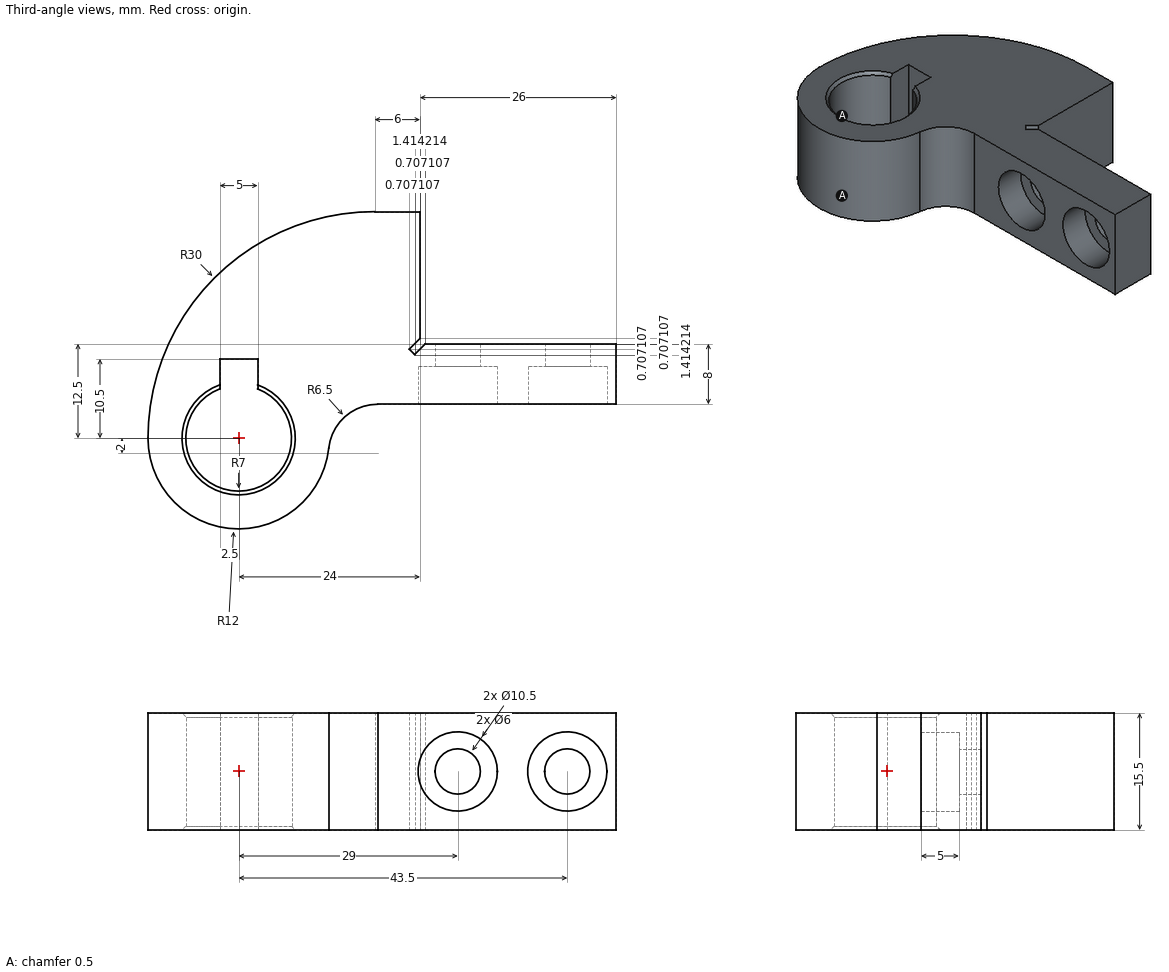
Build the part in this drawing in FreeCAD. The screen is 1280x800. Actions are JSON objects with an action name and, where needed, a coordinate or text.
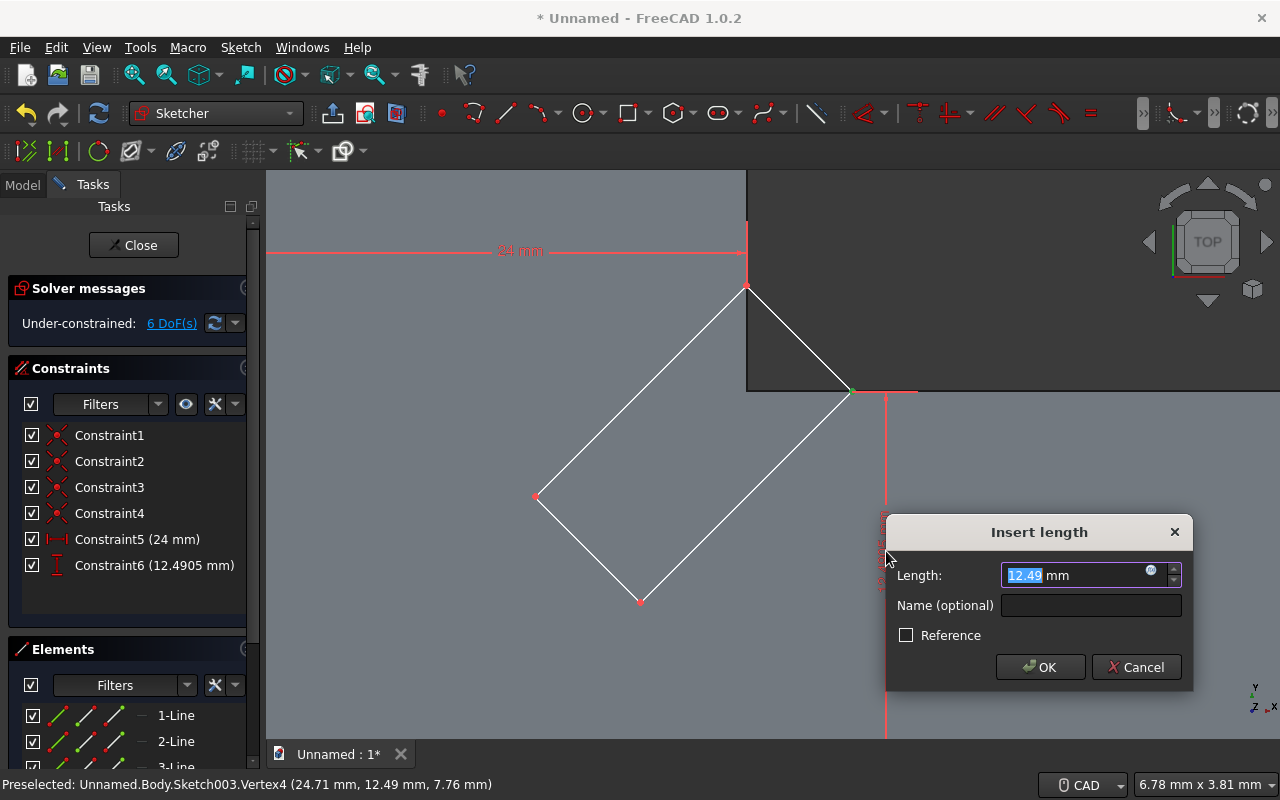
{"action": "type", "text": "12.5"}
{"action": "key", "text": "Return"}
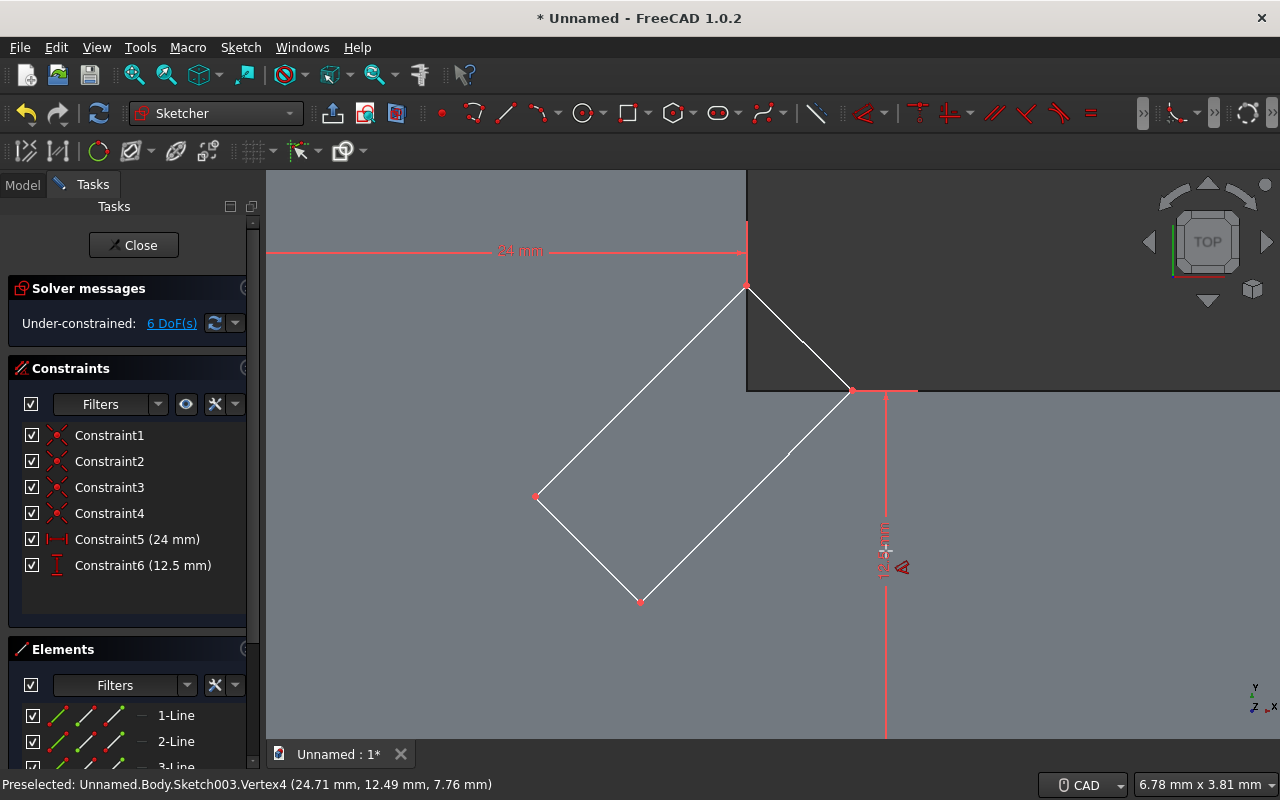
{"action": "left_click", "coordinate": [567, 529]}
{"action": "left_click", "coordinate": [588, 637]}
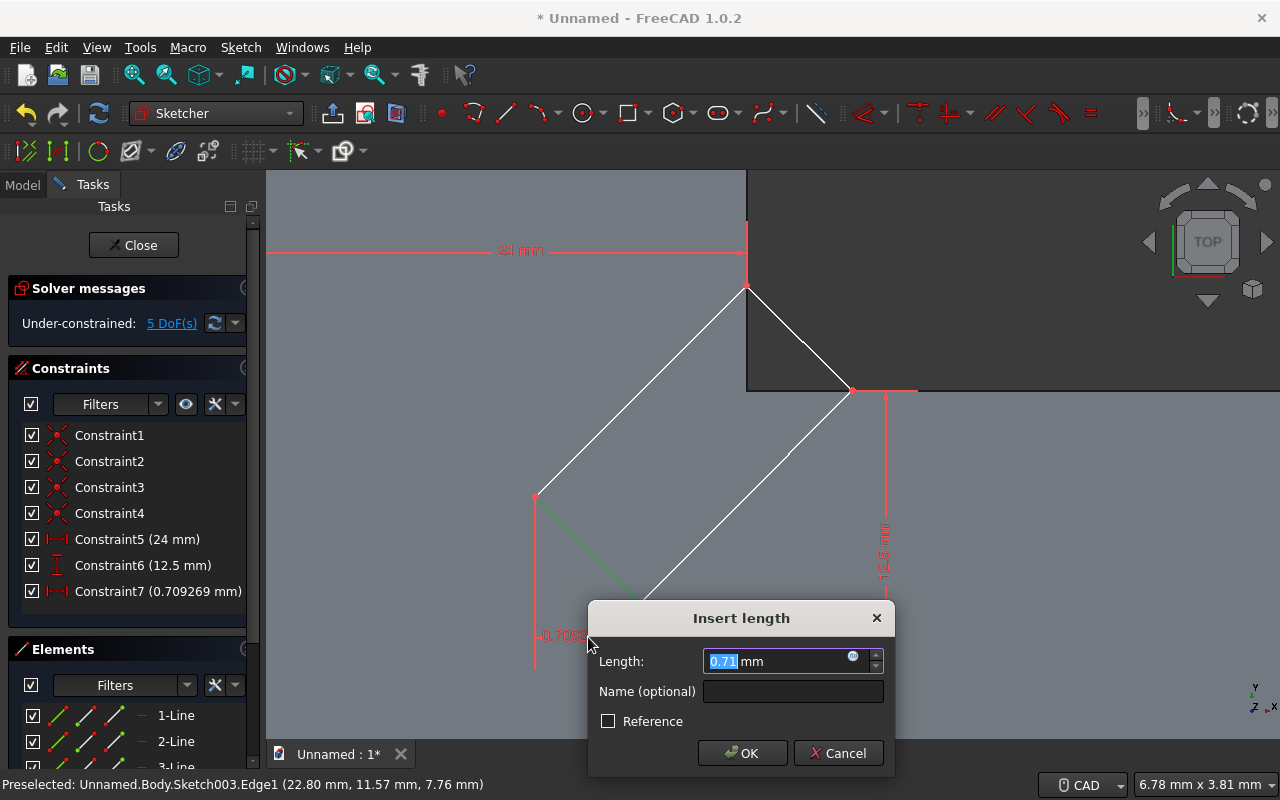
{"action": "type", "text": "0.707107"}
{"action": "key", "text": "Return"}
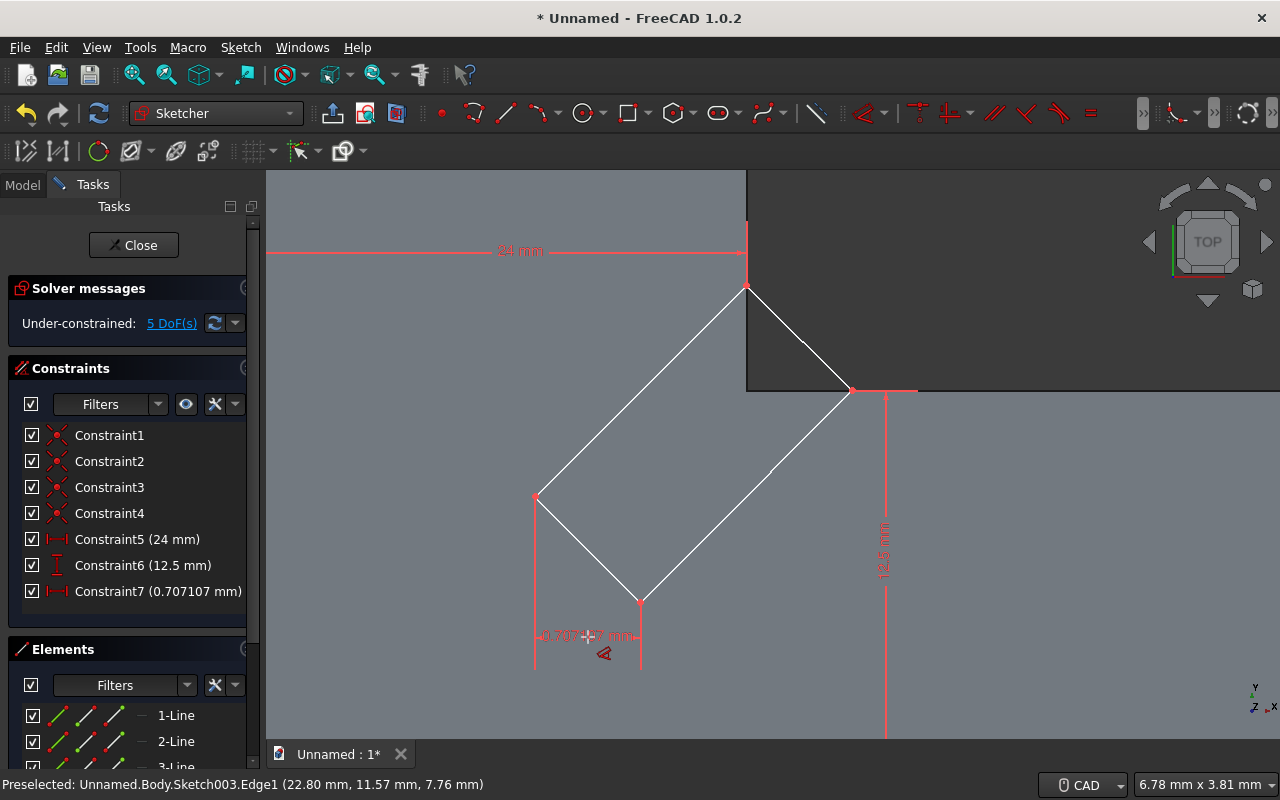
{"action": "left_click", "coordinate": [567, 529]}
{"action": "left_click", "coordinate": [501, 550]}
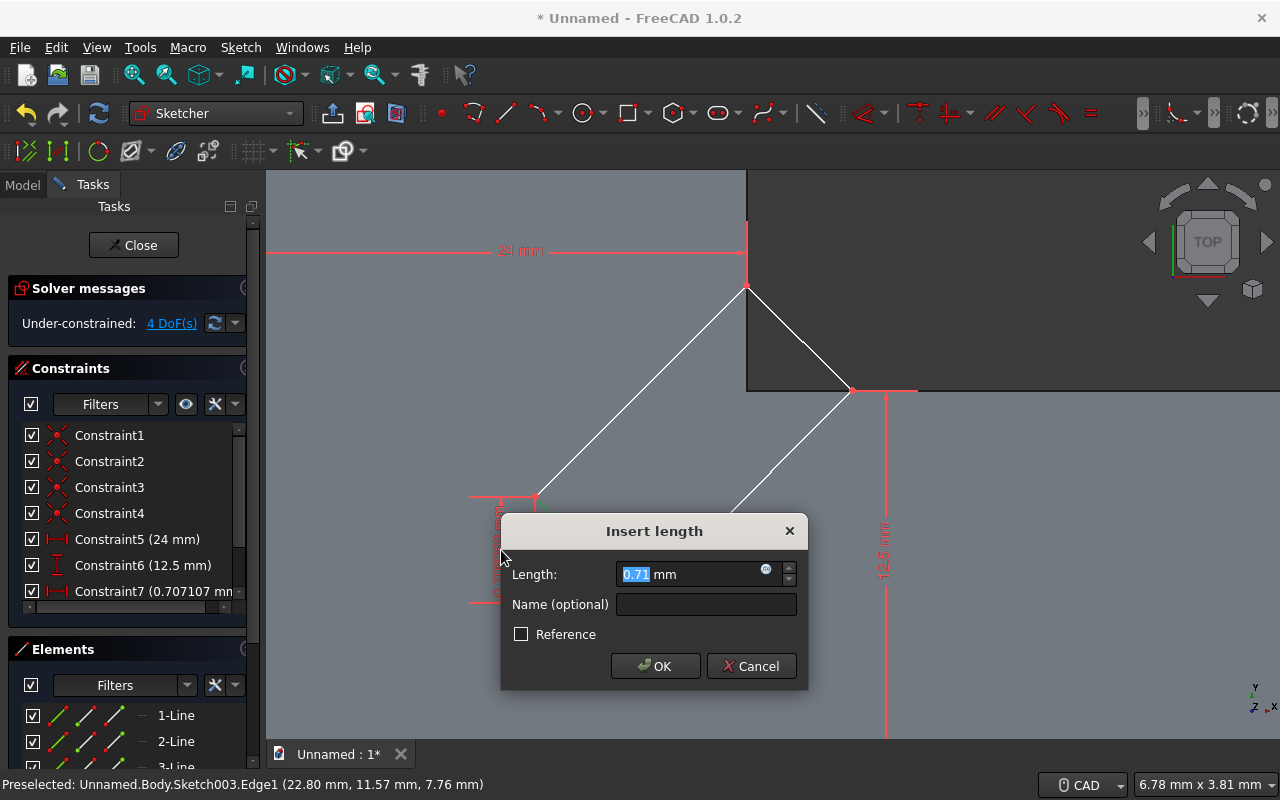
{"action": "type", "text": "0.707107"}
{"action": "key", "text": "Return"}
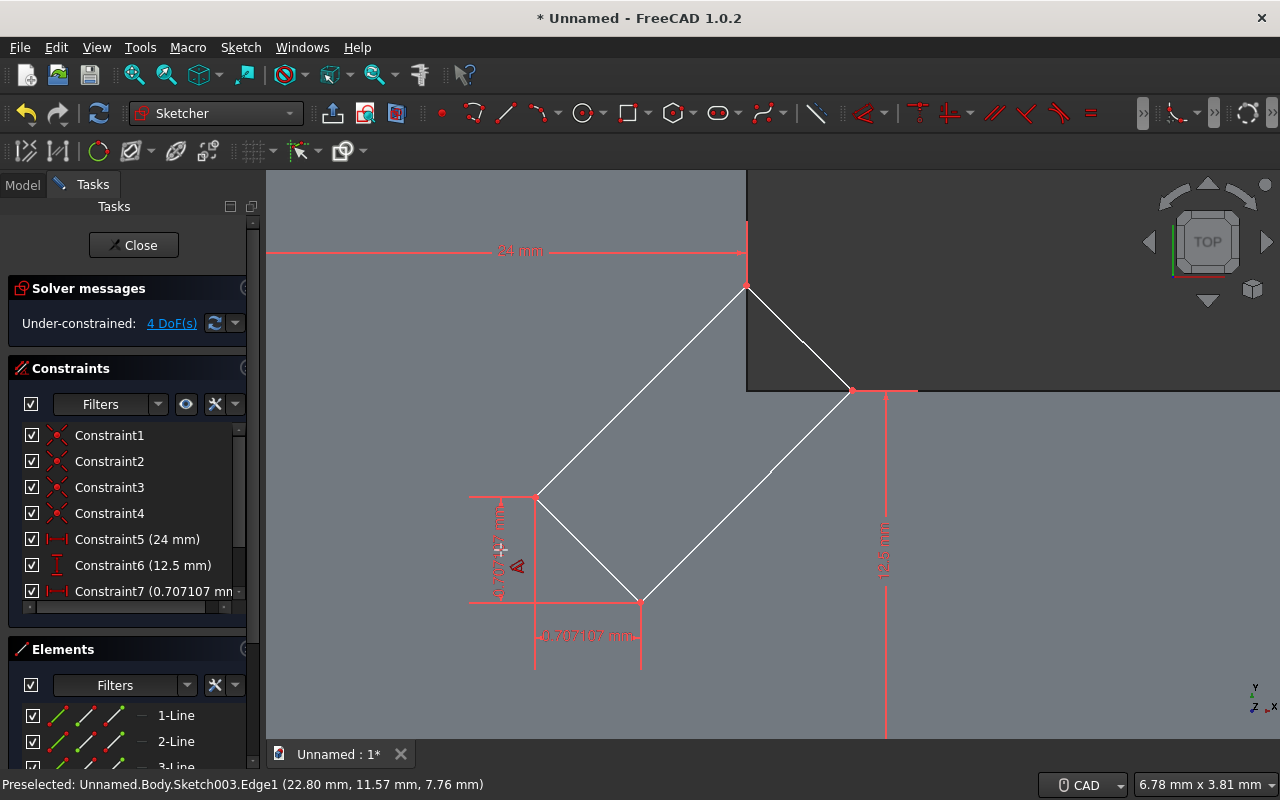
{"action": "left_click", "coordinate": [704, 539]}
{"action": "left_click", "coordinate": [746, 637]}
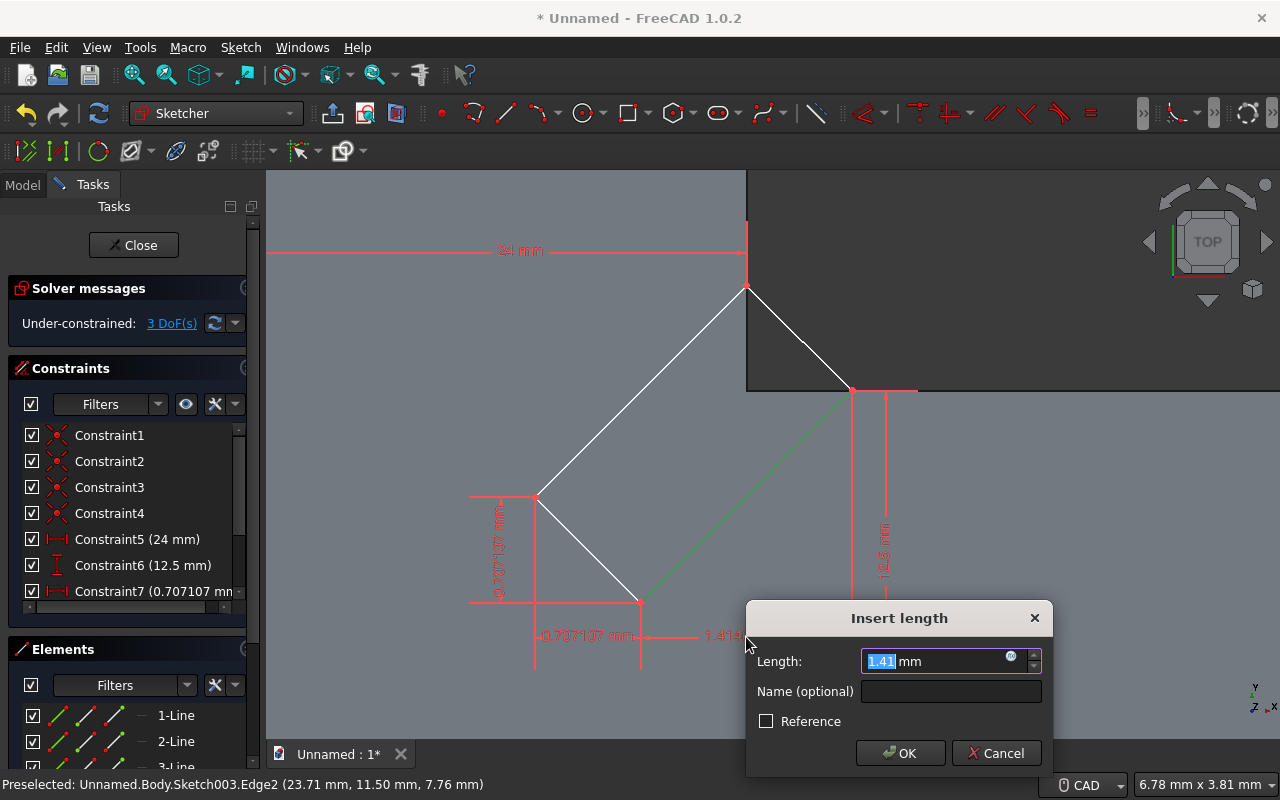
{"action": "type", "text": "1.414214"}
{"action": "key", "text": "Return"}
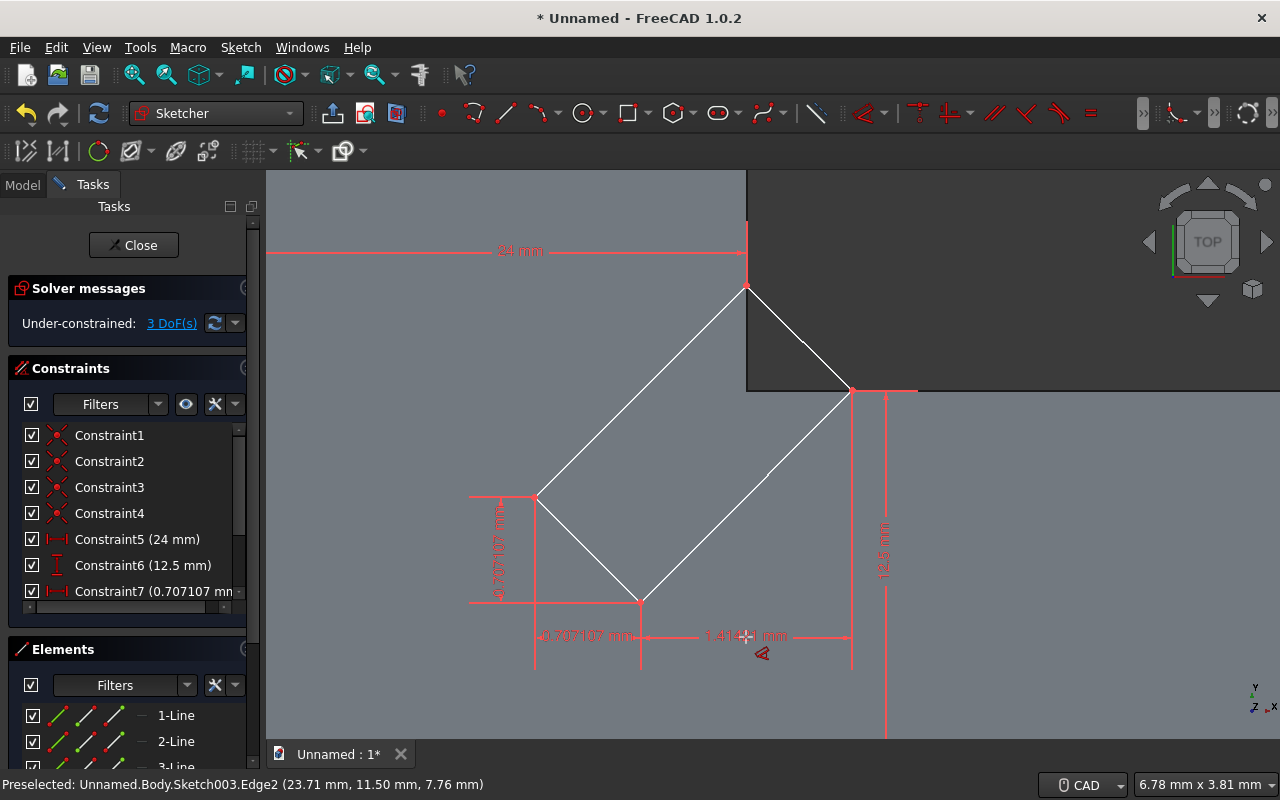
{"action": "left_click", "coordinate": [704, 539]}
{"action": "left_click", "coordinate": [886, 497]}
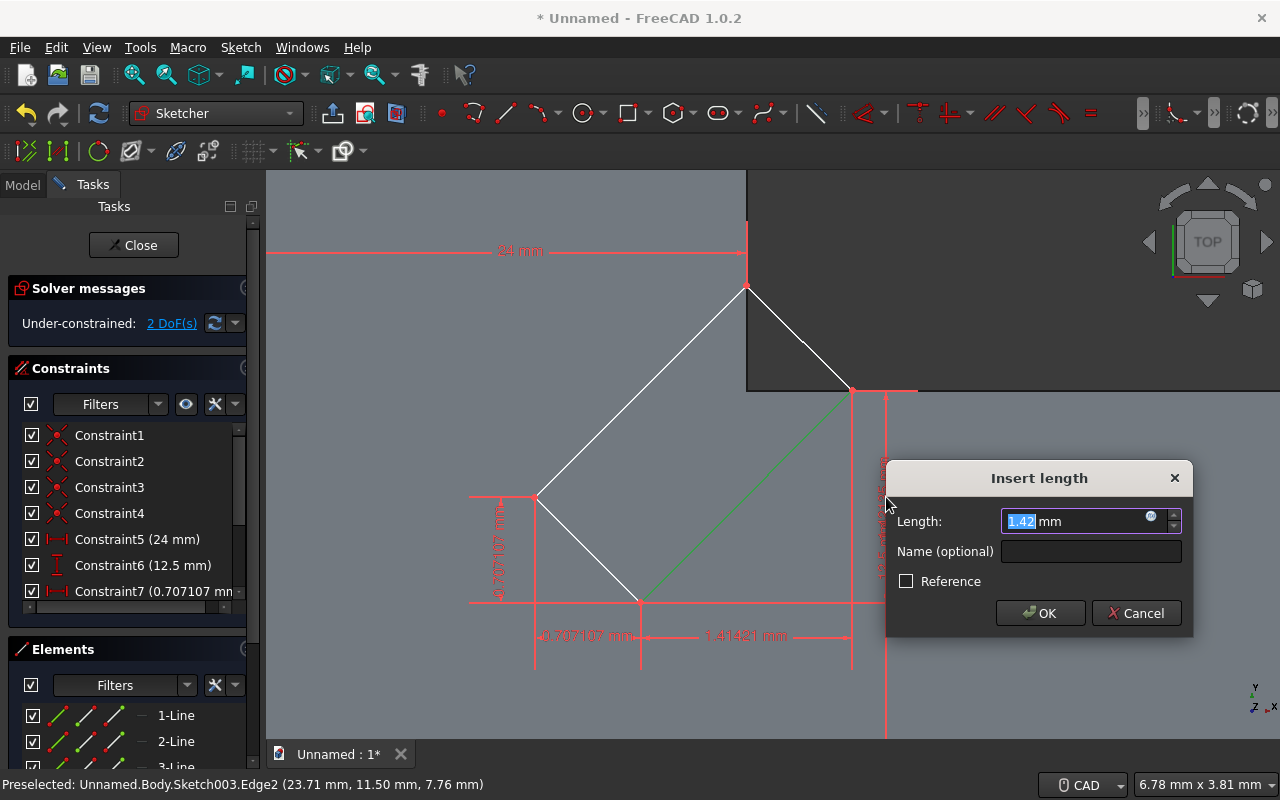
{"action": "type", "text": "1.414214"}
{"action": "key", "text": "Return"}